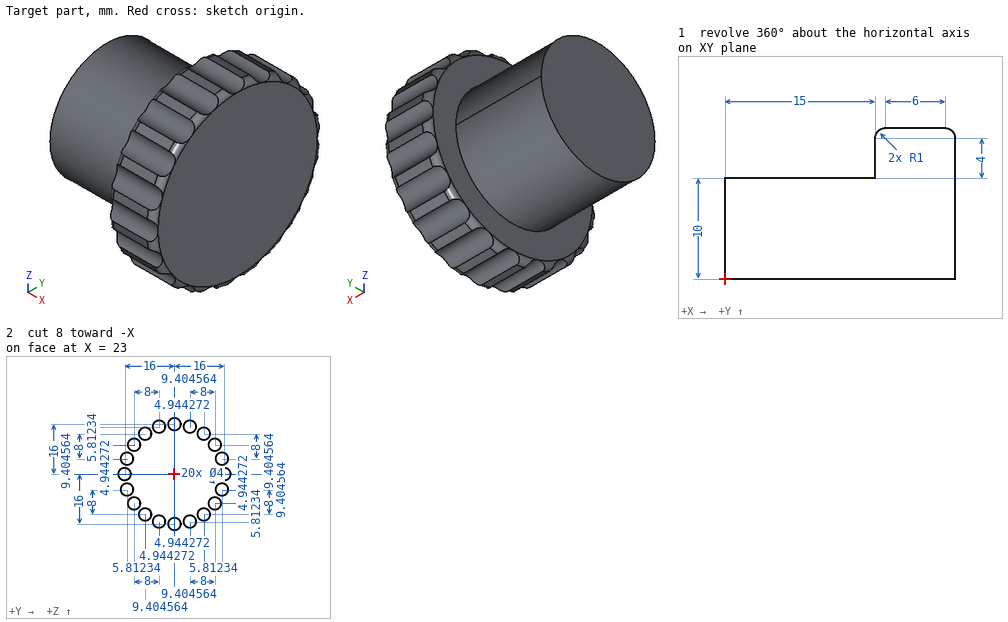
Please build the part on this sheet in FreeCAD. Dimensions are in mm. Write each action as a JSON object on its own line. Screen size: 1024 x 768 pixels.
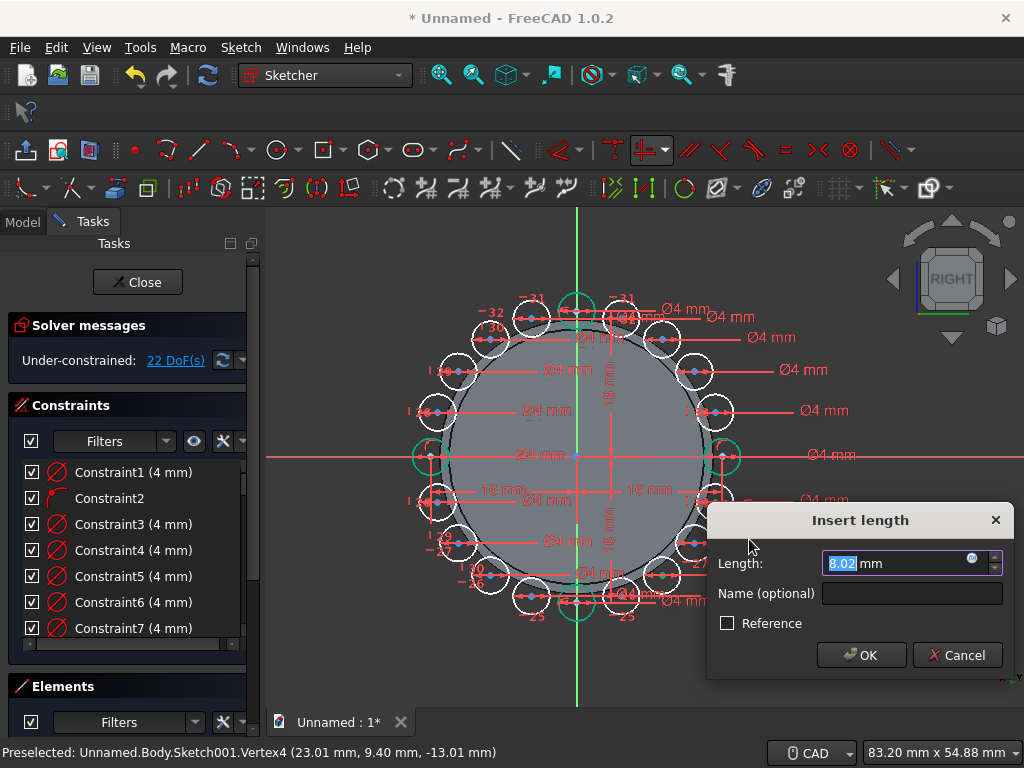
{"action": "type", "text": "8"}
{"action": "key", "text": "Return"}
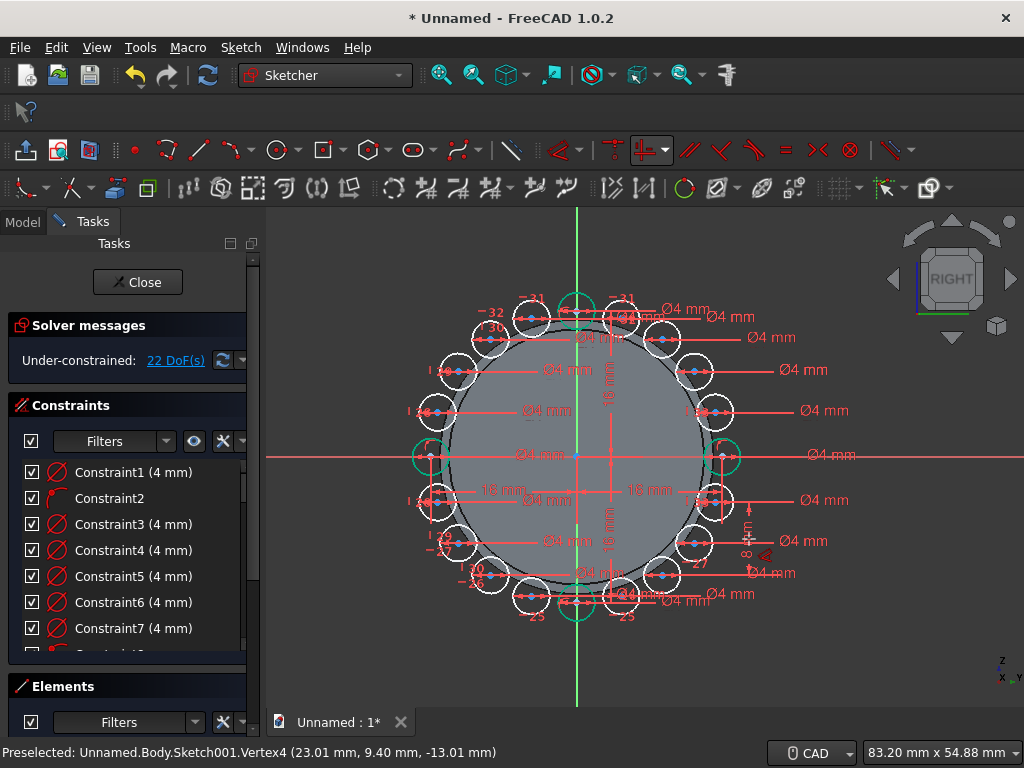
{"action": "left_click", "coordinate": [694, 543]}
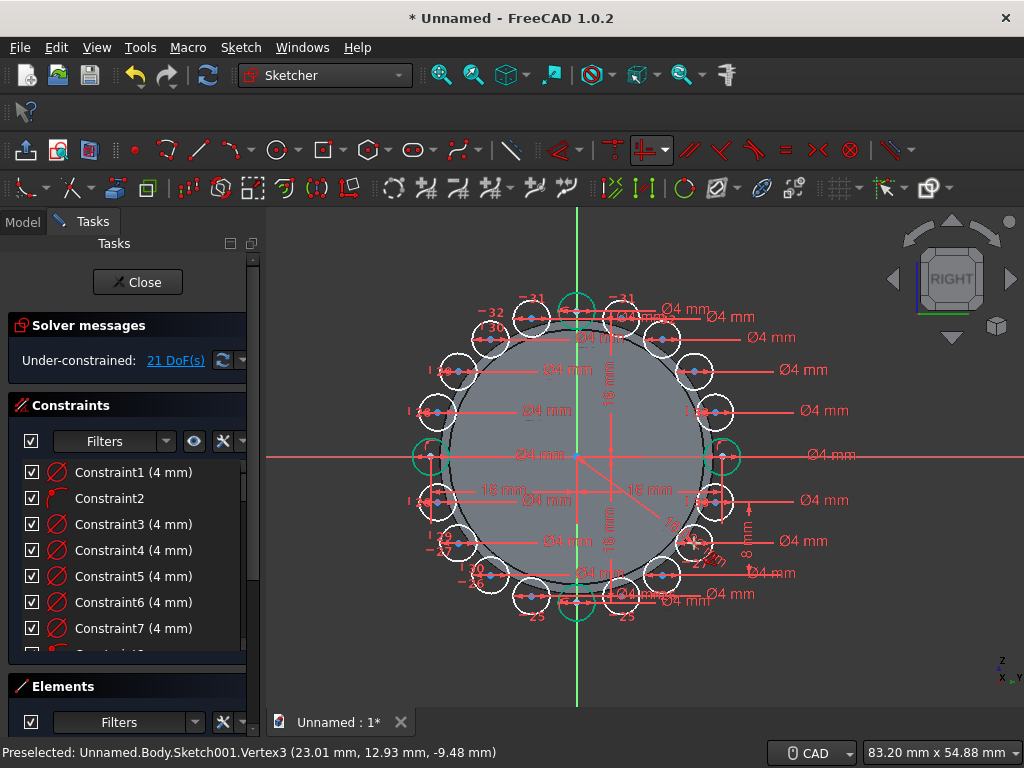
{"action": "left_click", "coordinate": [621, 596]}
{"action": "left_click", "coordinate": [658, 630]}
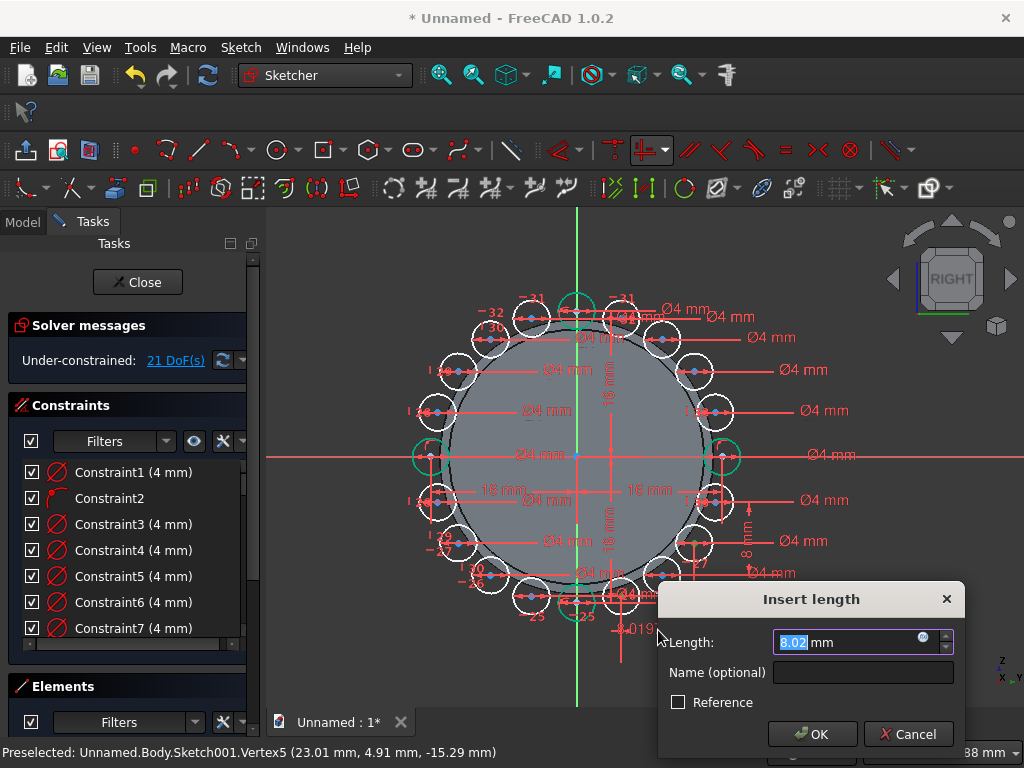
{"action": "type", "text": "8"}
{"action": "key", "text": "Return"}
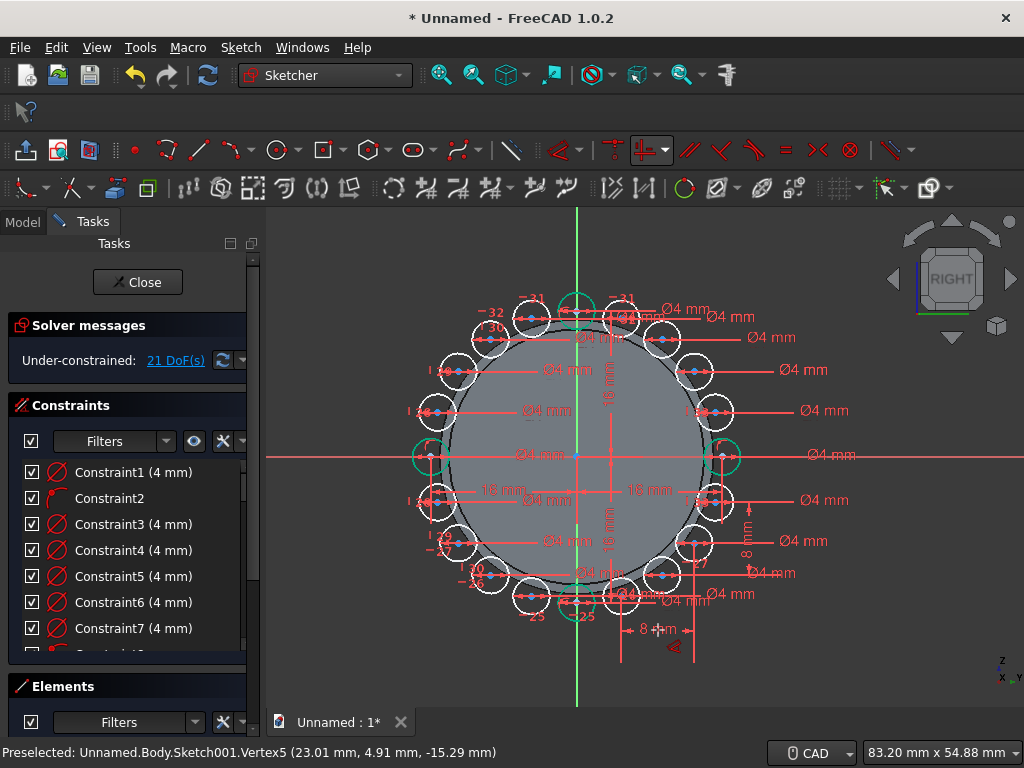
{"action": "left_click", "coordinate": [531, 596]}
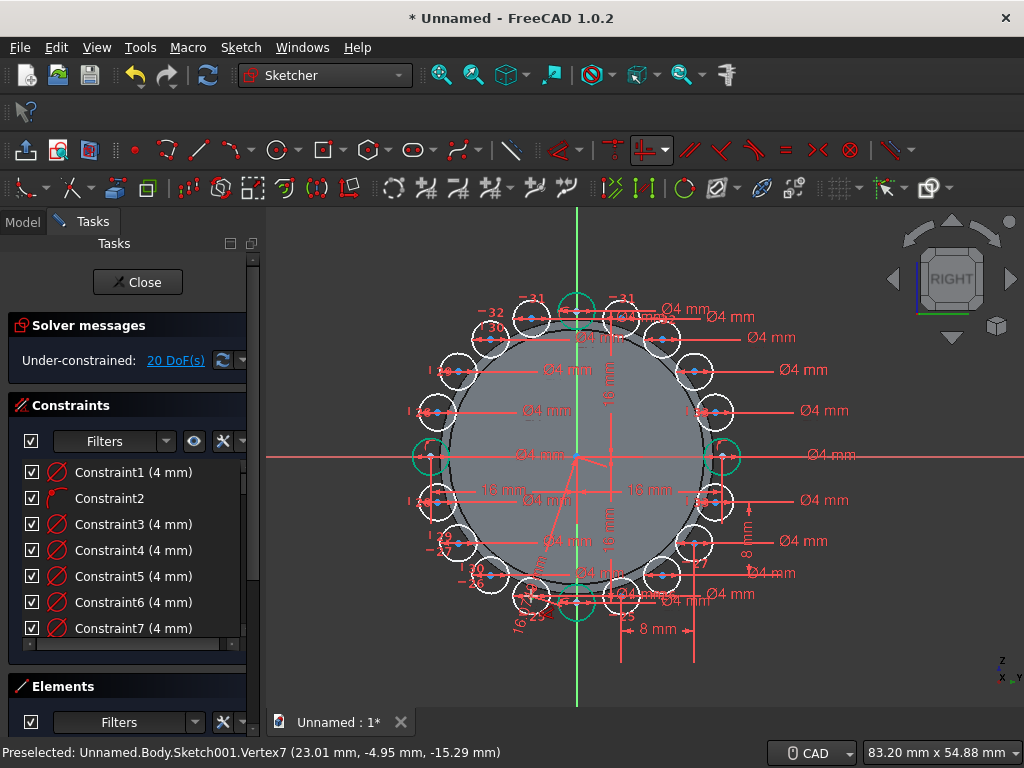
{"action": "left_click", "coordinate": [458, 543]}
{"action": "left_click", "coordinate": [495, 630]}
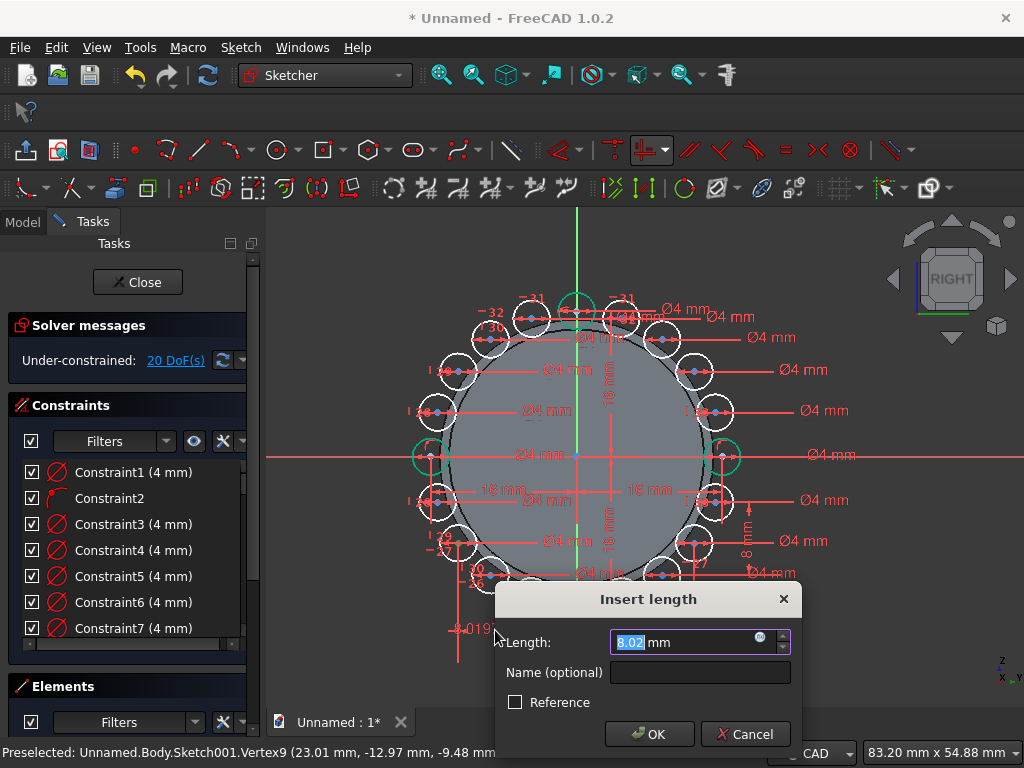
{"action": "type", "text": "8"}
{"action": "key", "text": "Return"}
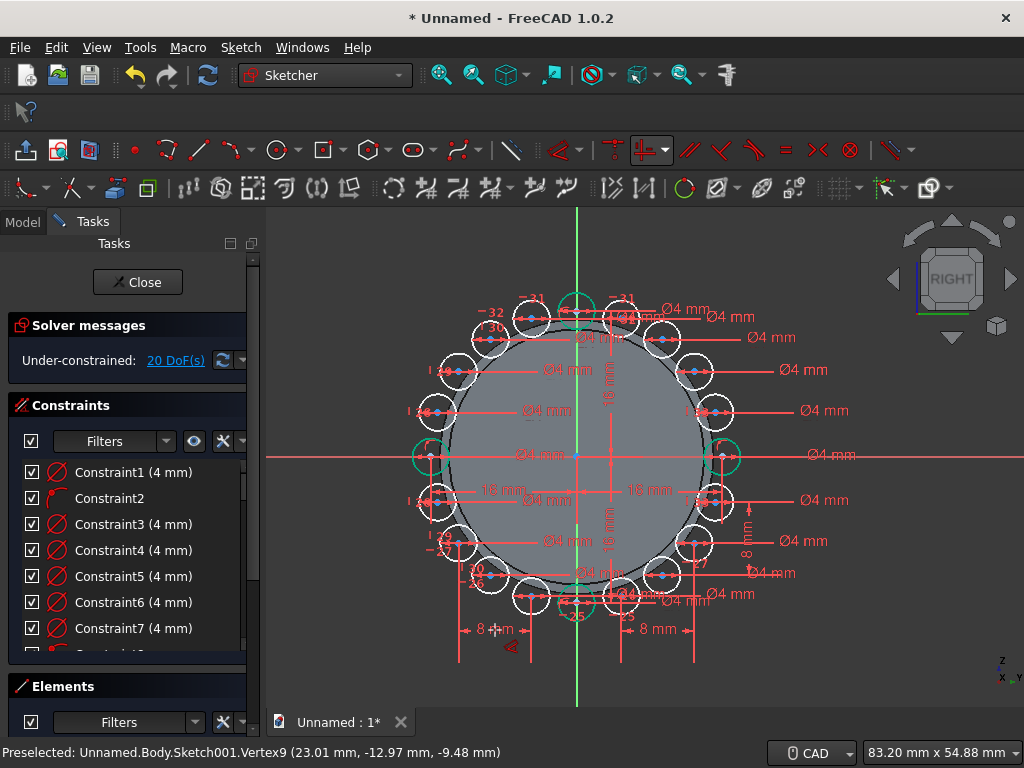
{"action": "left_click", "coordinate": [491, 575]}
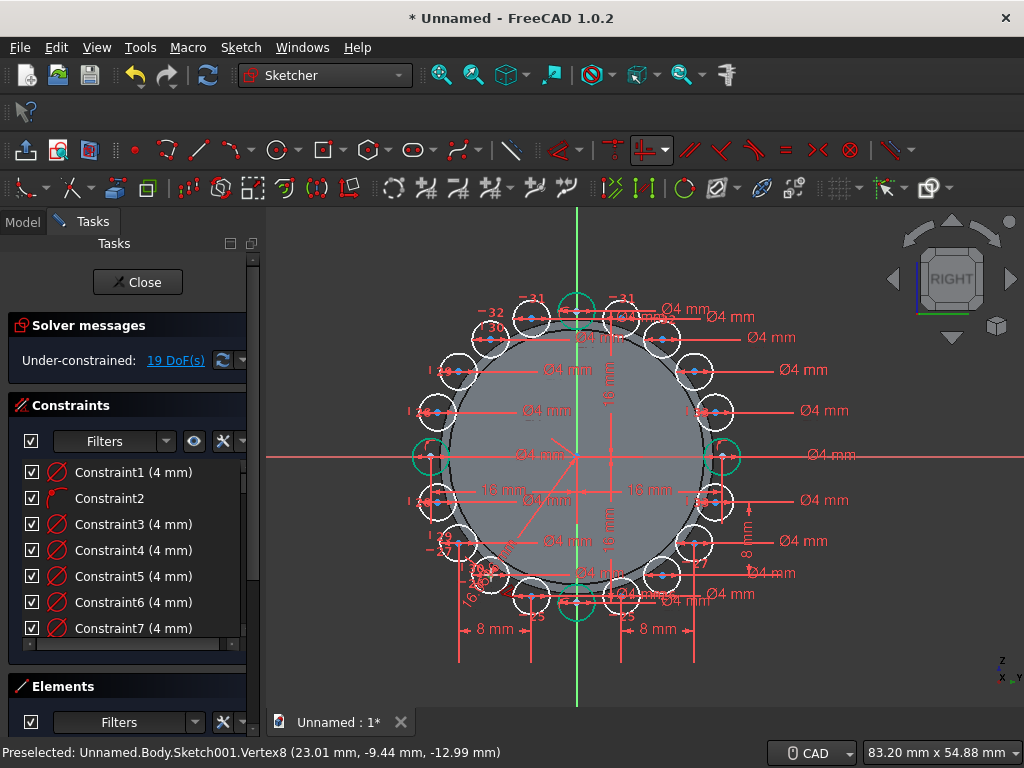
{"action": "left_click", "coordinate": [438, 502]}
{"action": "left_click", "coordinate": [404, 539]}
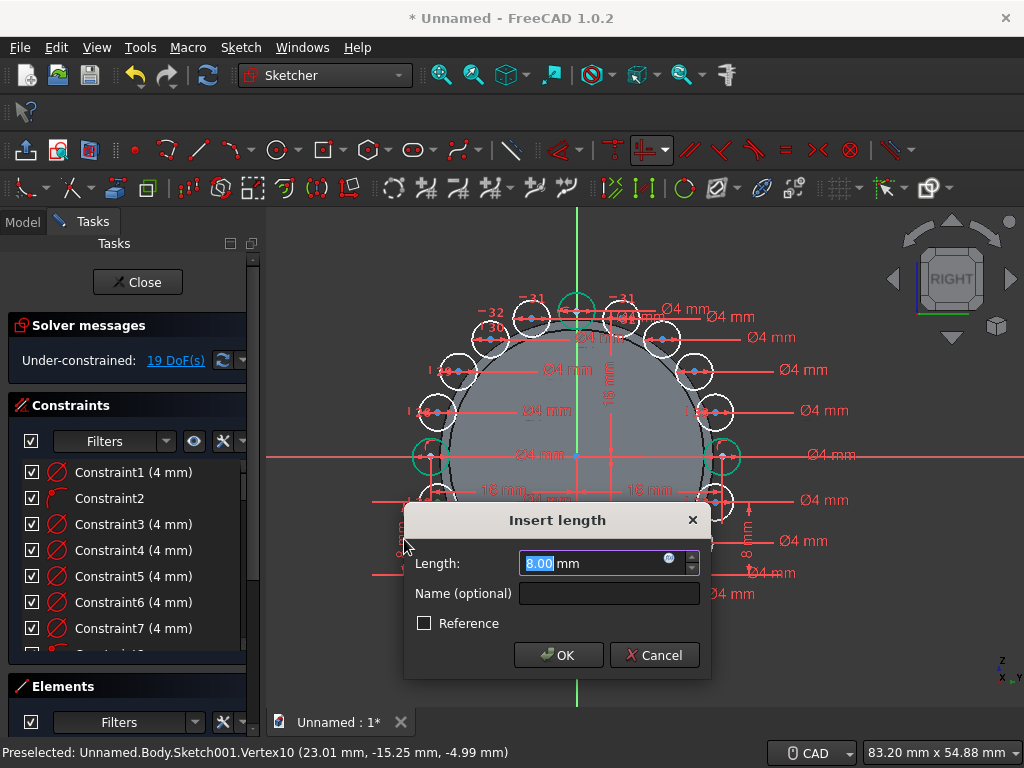
{"action": "type", "text": "8"}
{"action": "key", "text": "Return"}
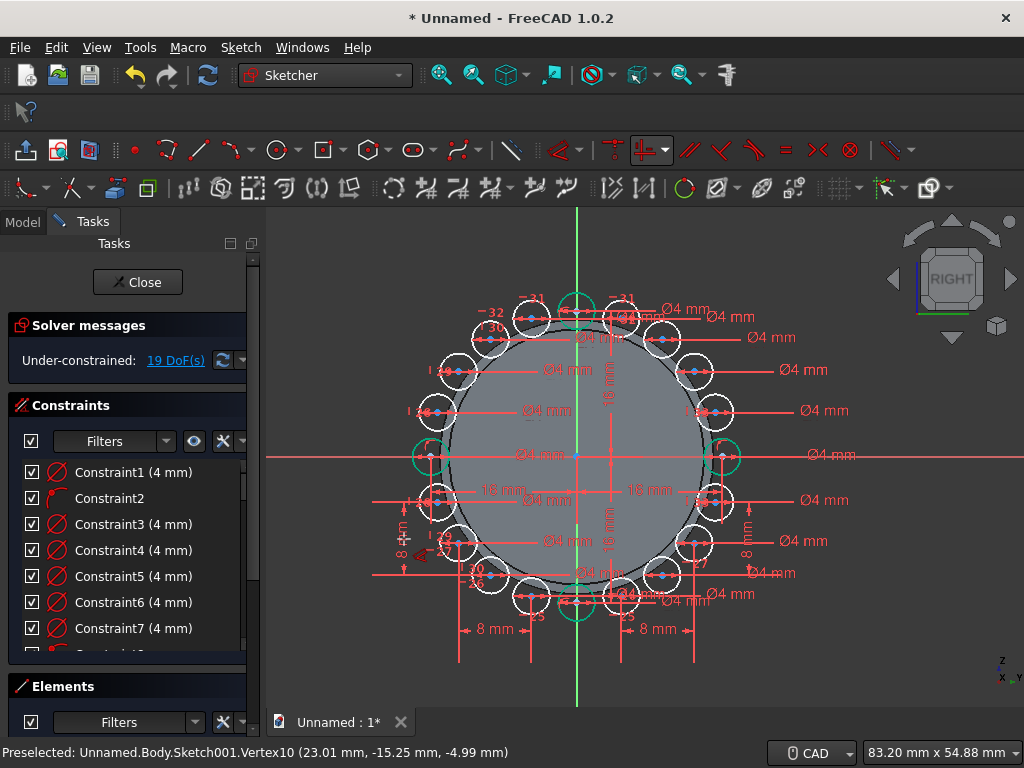
{"action": "left_click", "coordinate": [438, 413]}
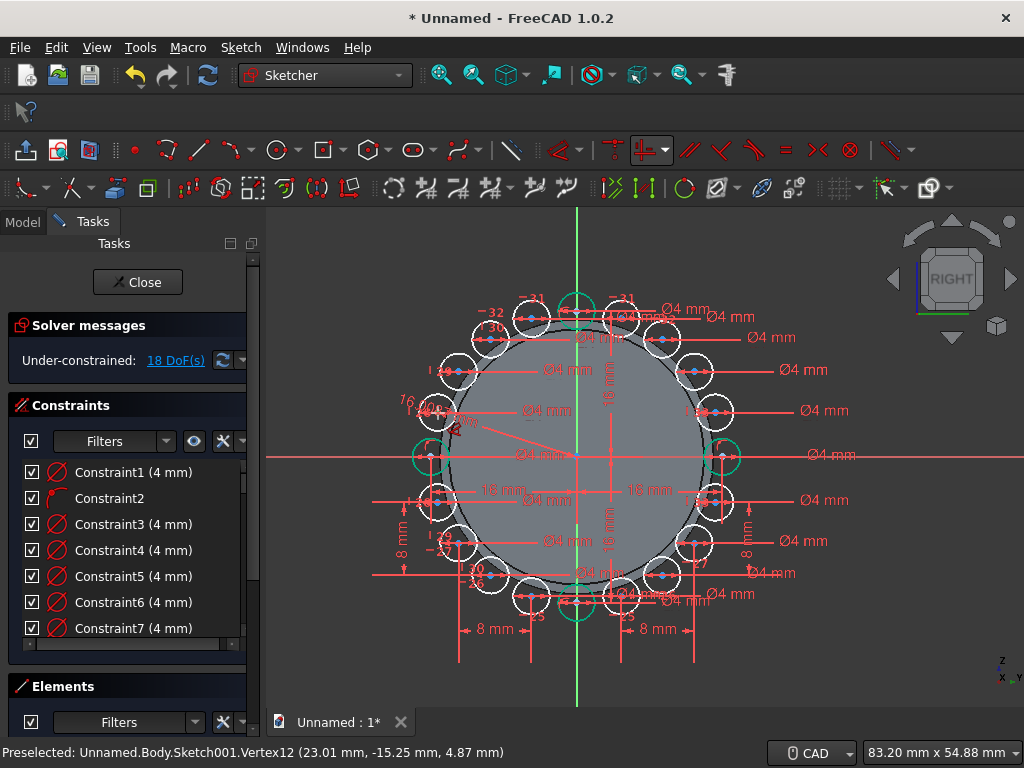
{"action": "left_click", "coordinate": [491, 340]}
{"action": "left_click", "coordinate": [404, 376]}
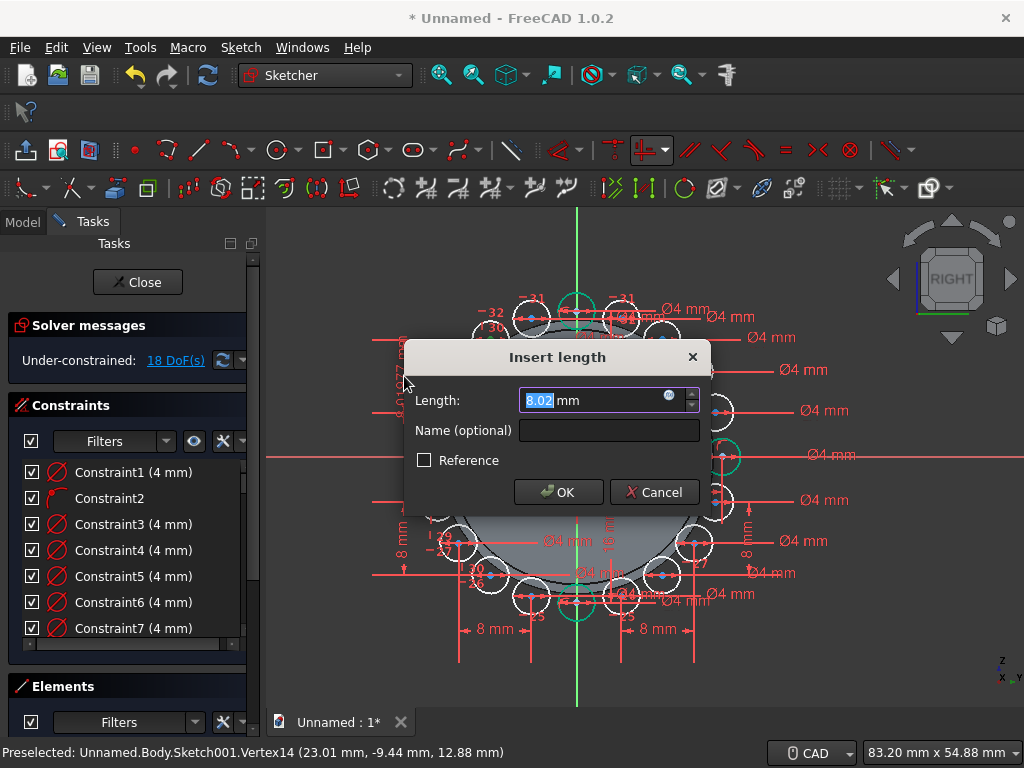
{"action": "type", "text": "8"}
{"action": "key", "text": "Return"}